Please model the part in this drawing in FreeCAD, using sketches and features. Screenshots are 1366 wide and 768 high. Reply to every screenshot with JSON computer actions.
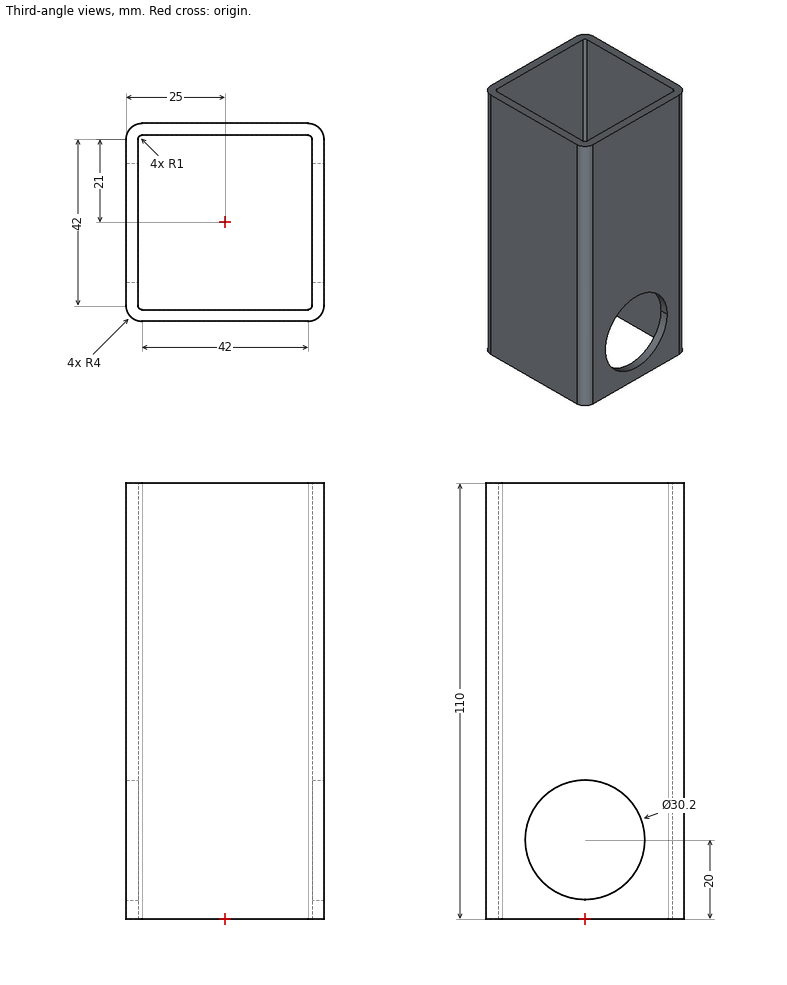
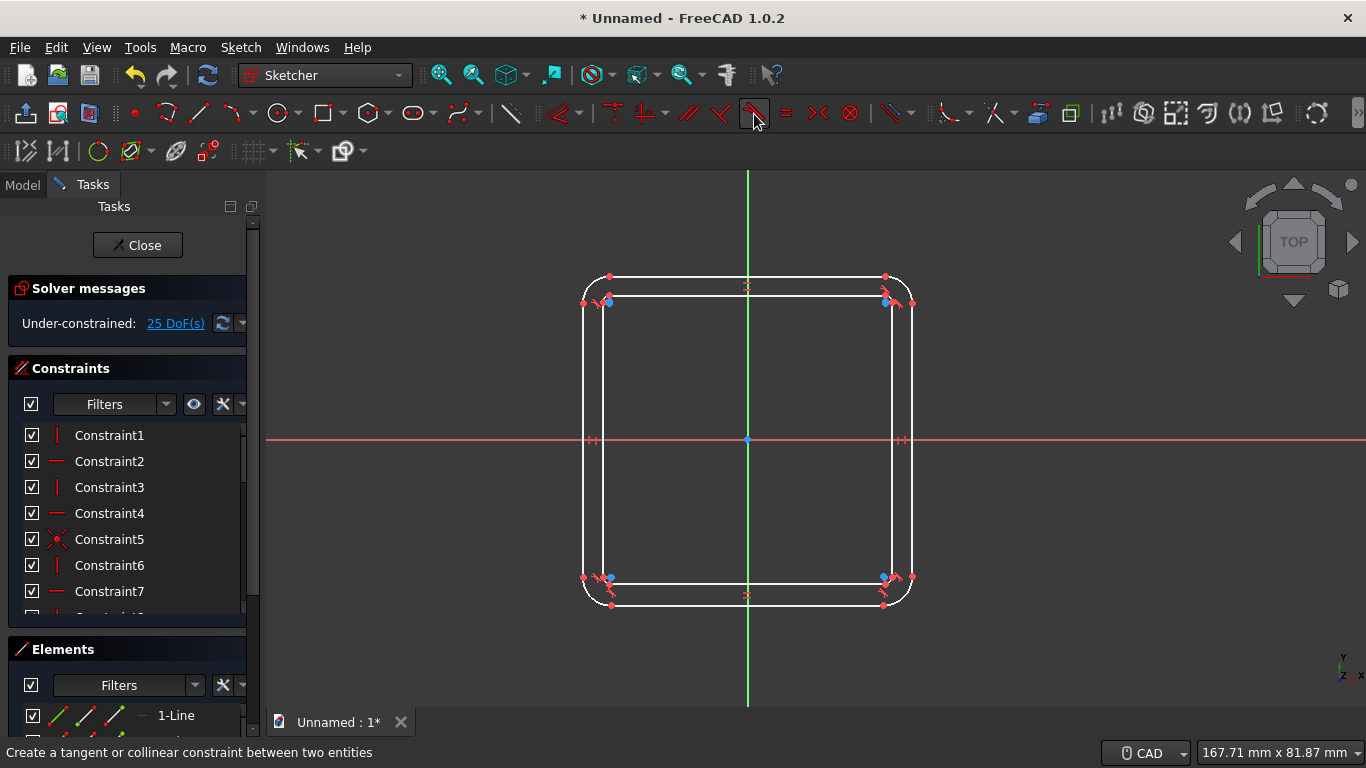
{"action": "left_click", "coordinate": [803, 277]}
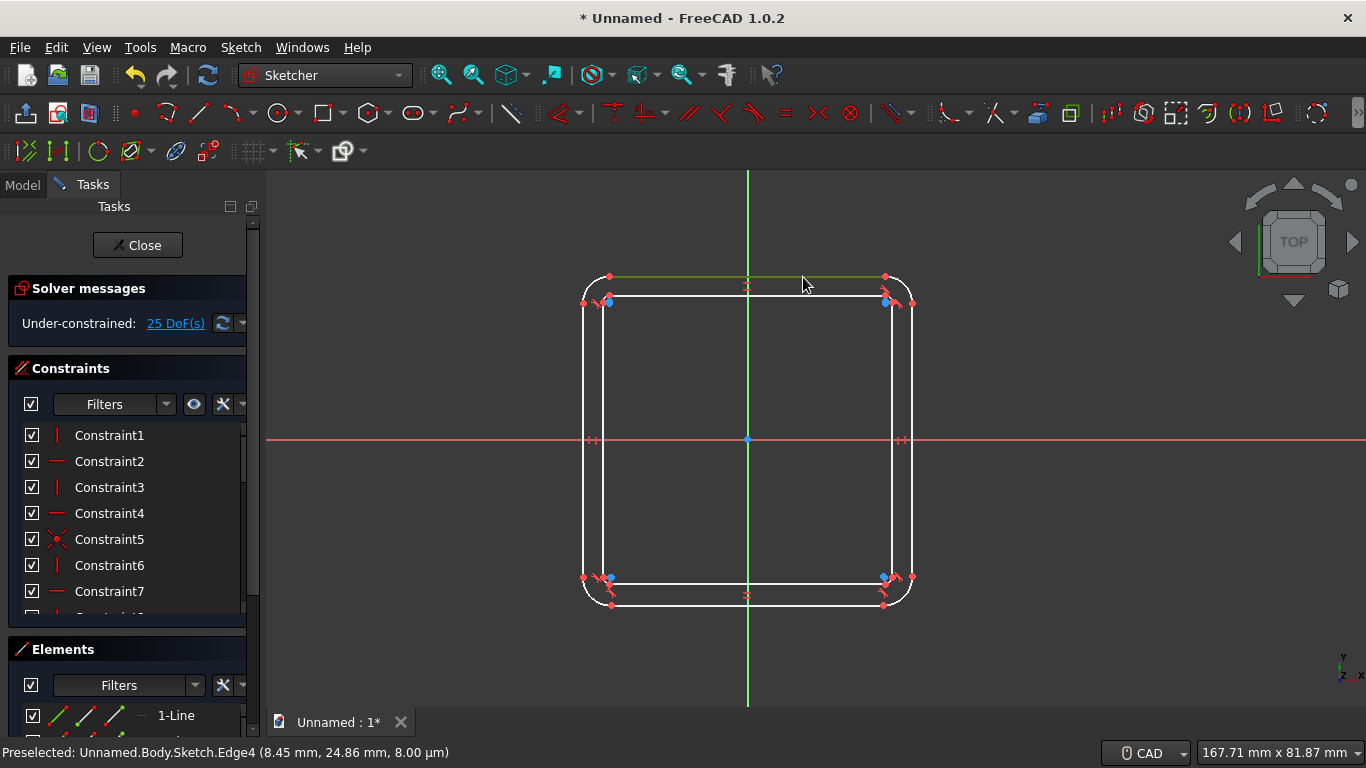
{"action": "left_click", "coordinate": [597, 280]}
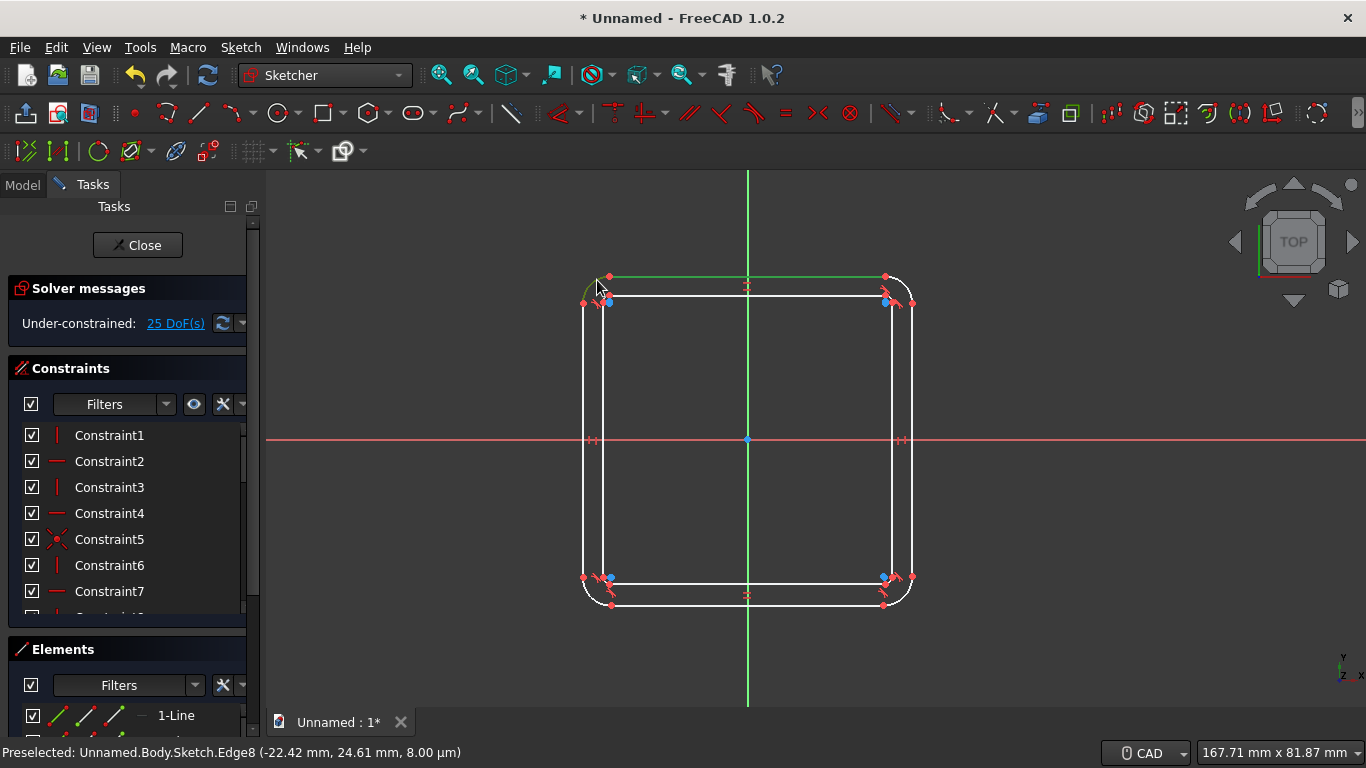
{"action": "left_click", "coordinate": [754, 114]}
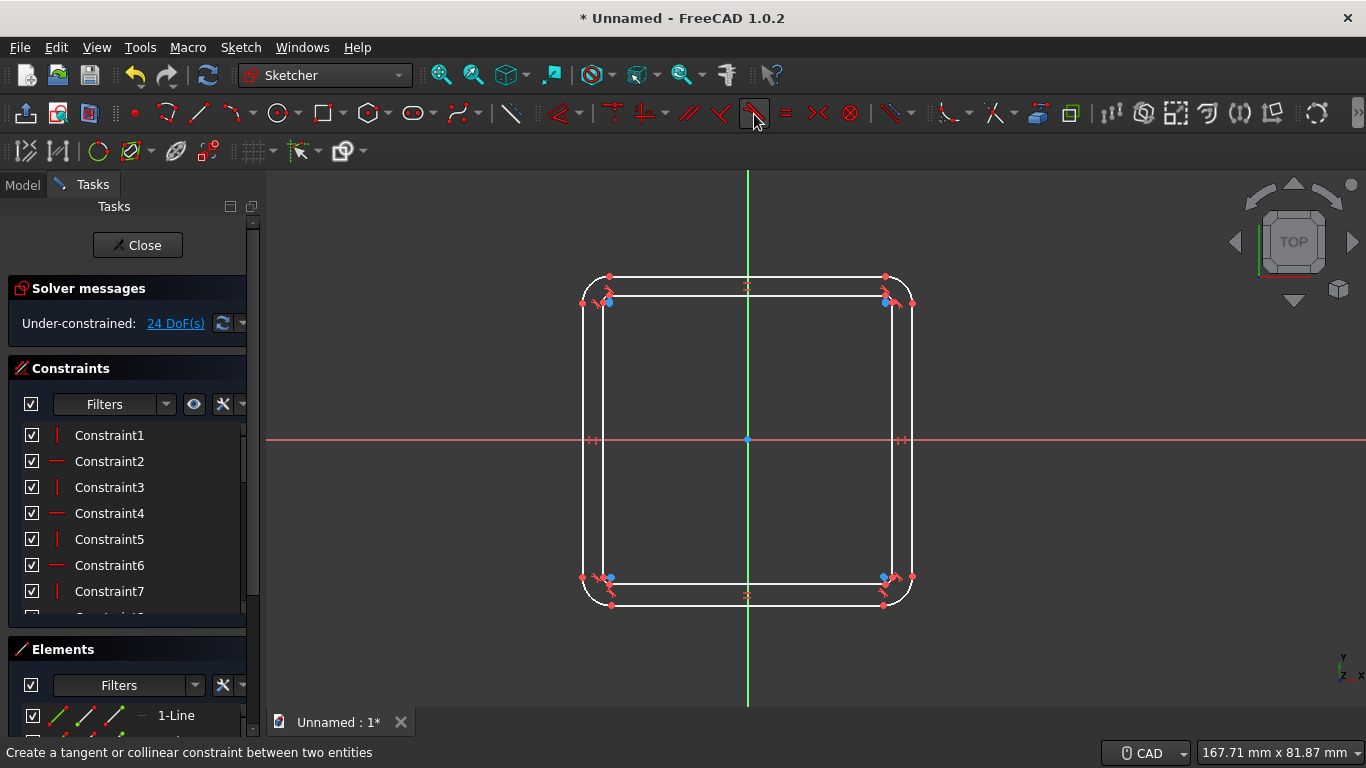
{"action": "left_click", "coordinate": [603, 495]}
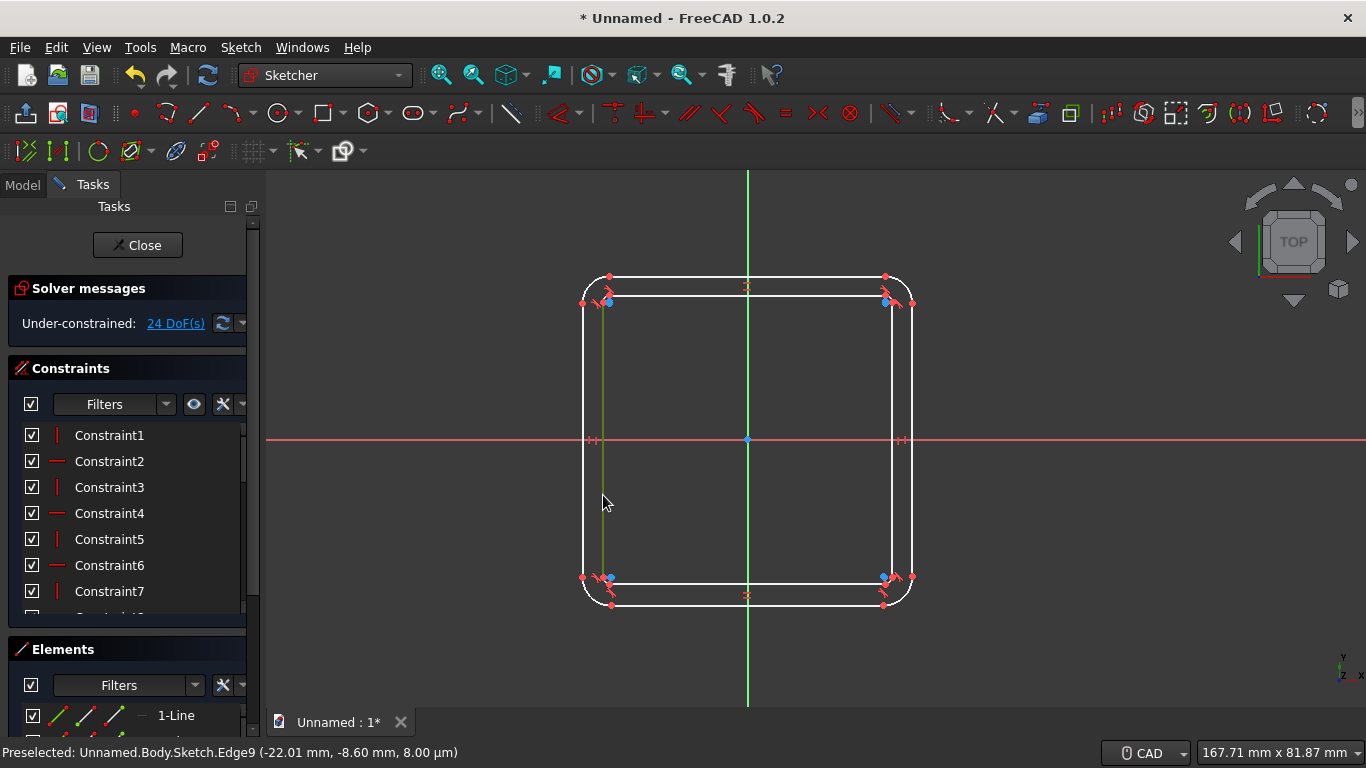
{"action": "scroll", "coordinate": [605, 297], "scroll_direction": "up", "scroll_amount": 5}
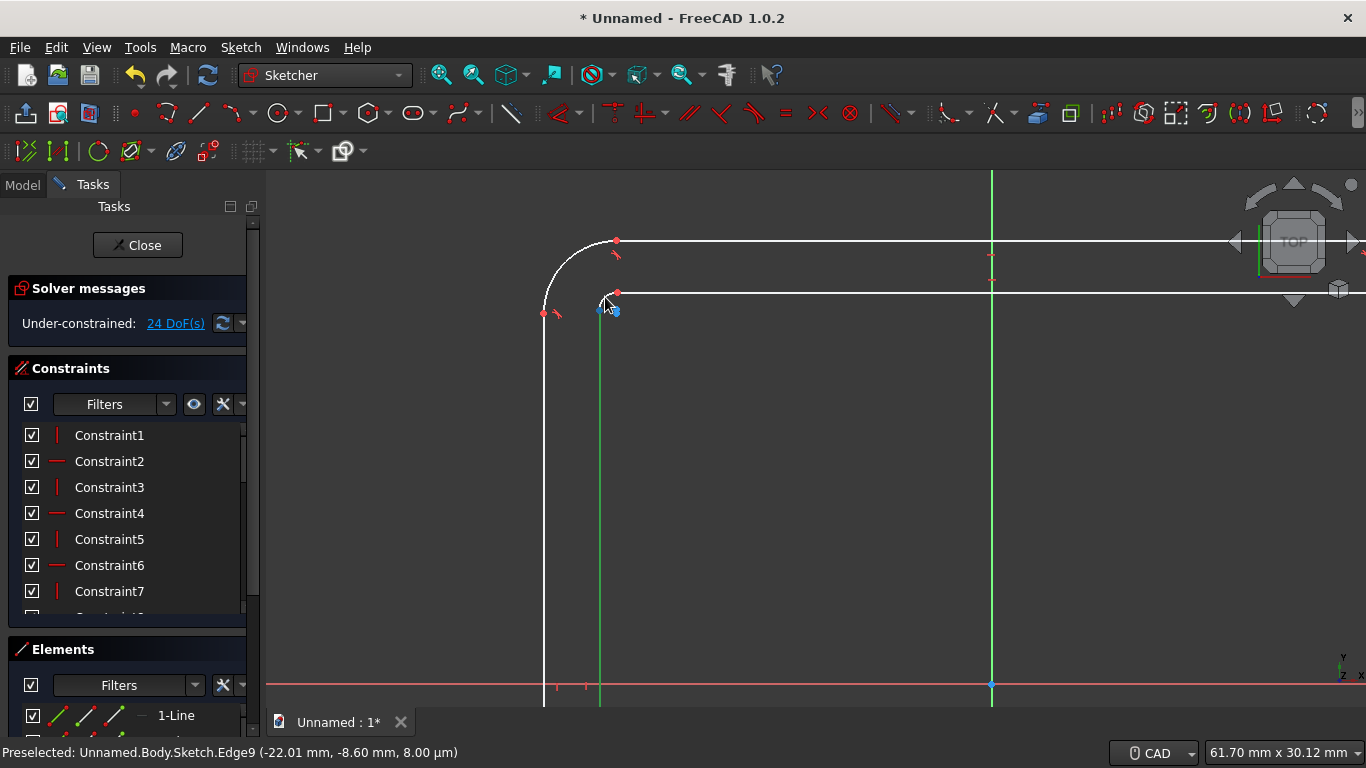
{"action": "left_click", "coordinate": [604, 298]}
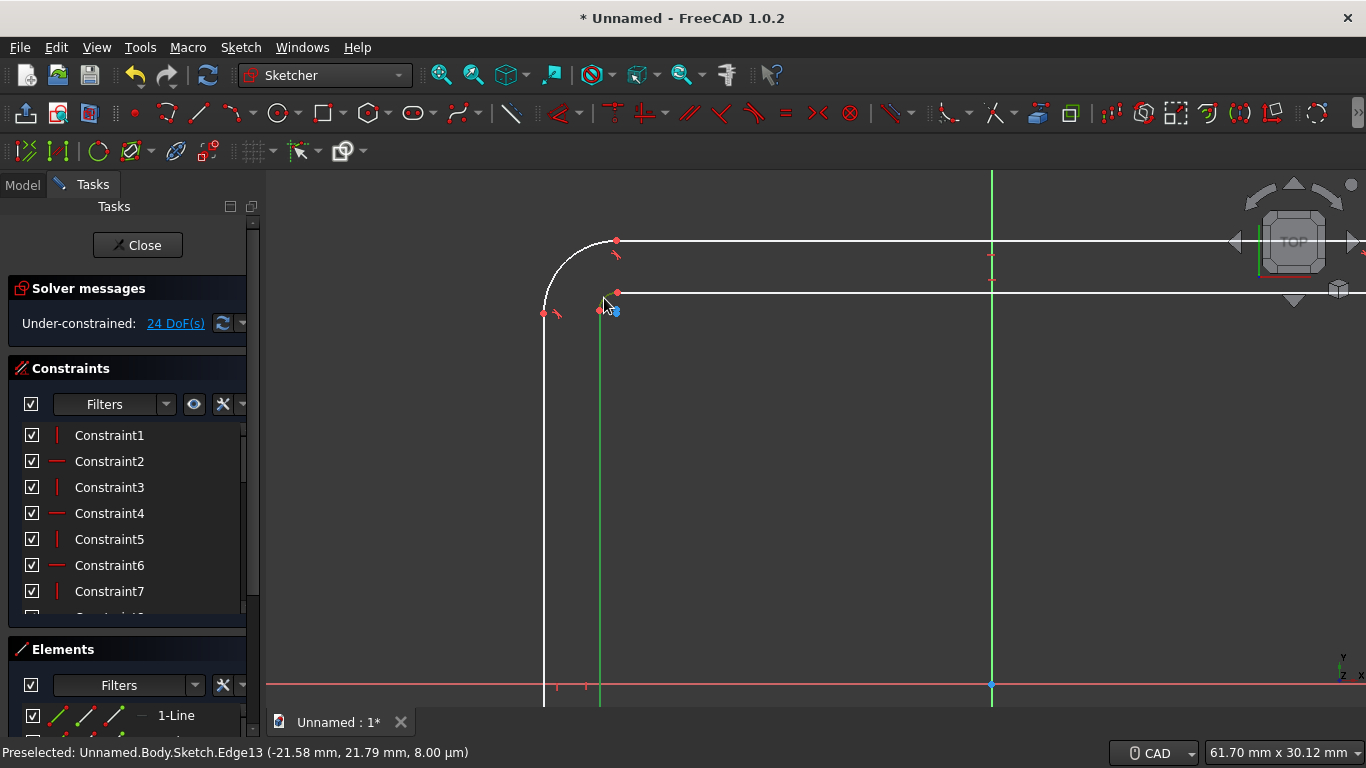
{"action": "left_click", "coordinate": [754, 114]}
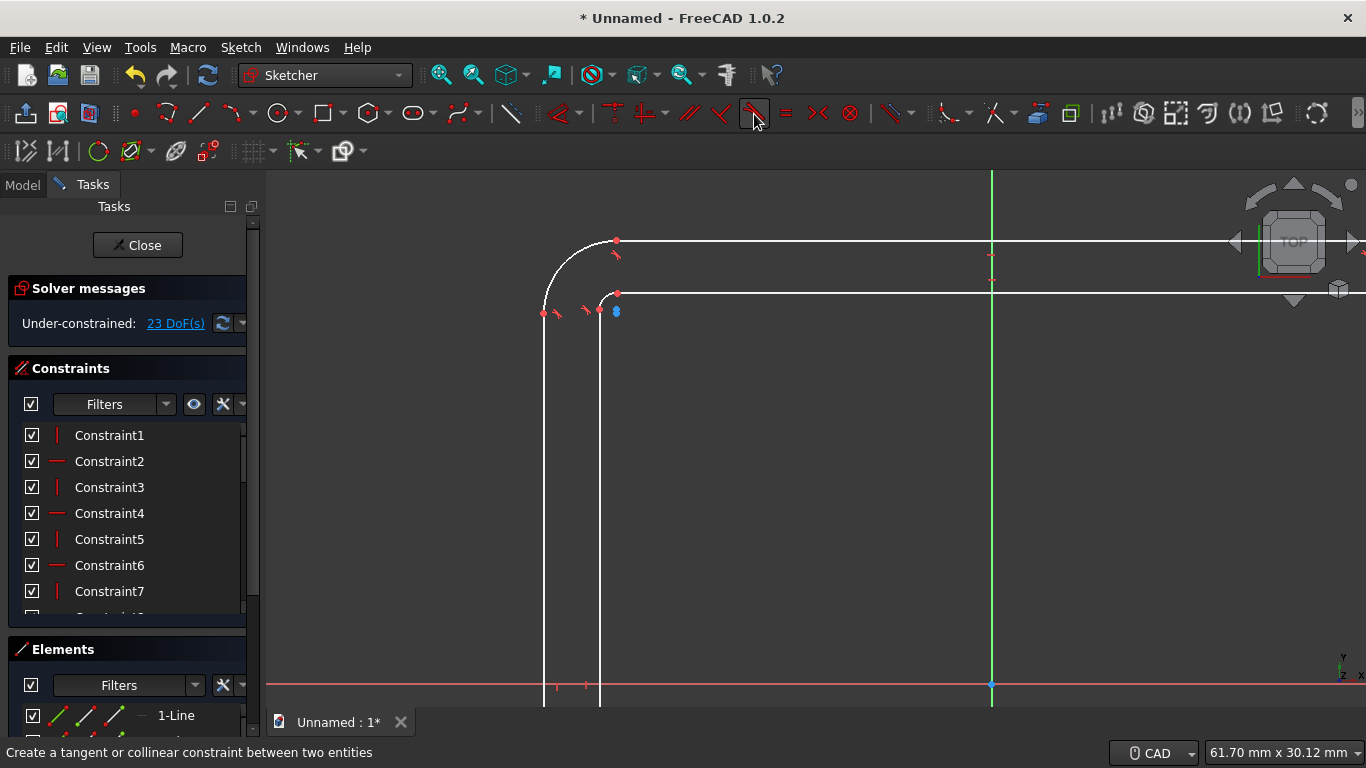
{"action": "left_click", "coordinate": [600, 534]}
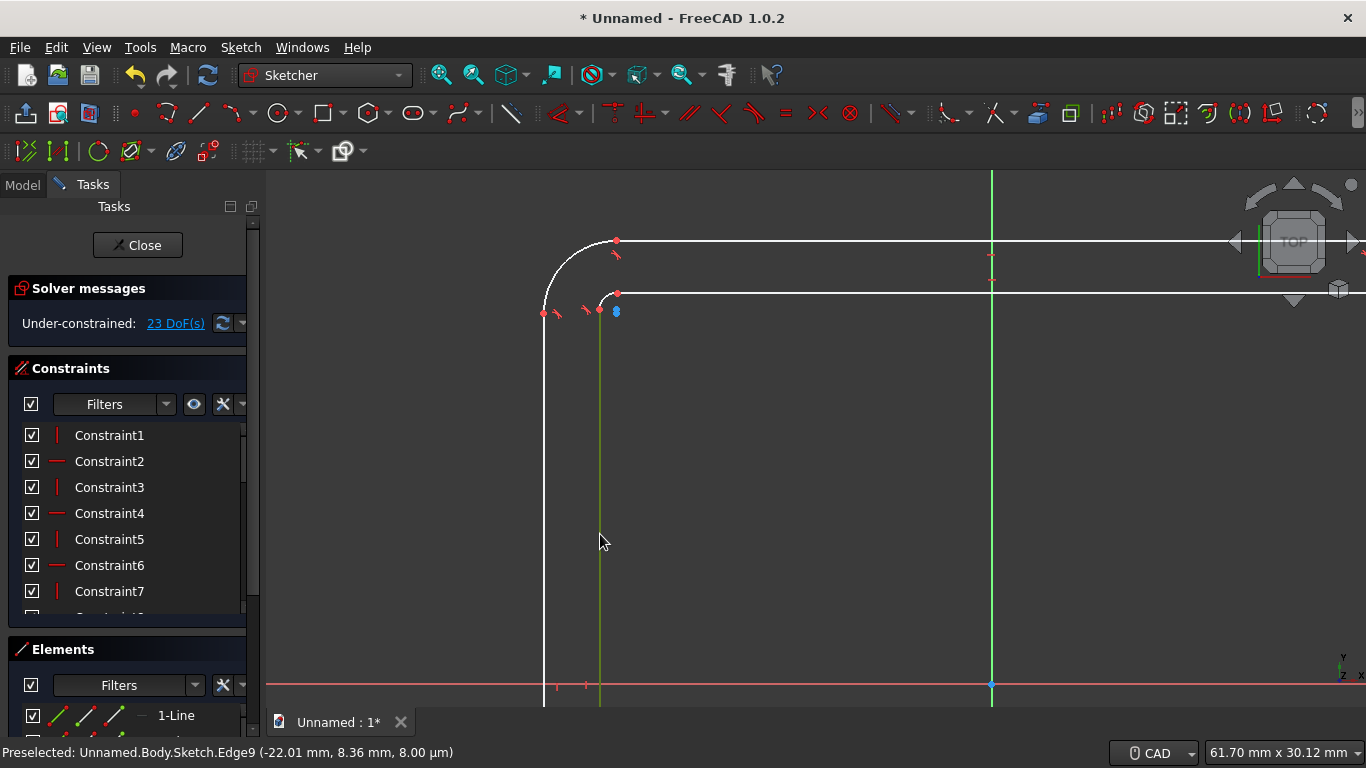
{"action": "scroll", "coordinate": [605, 296], "scroll_direction": "down", "scroll_amount": 5}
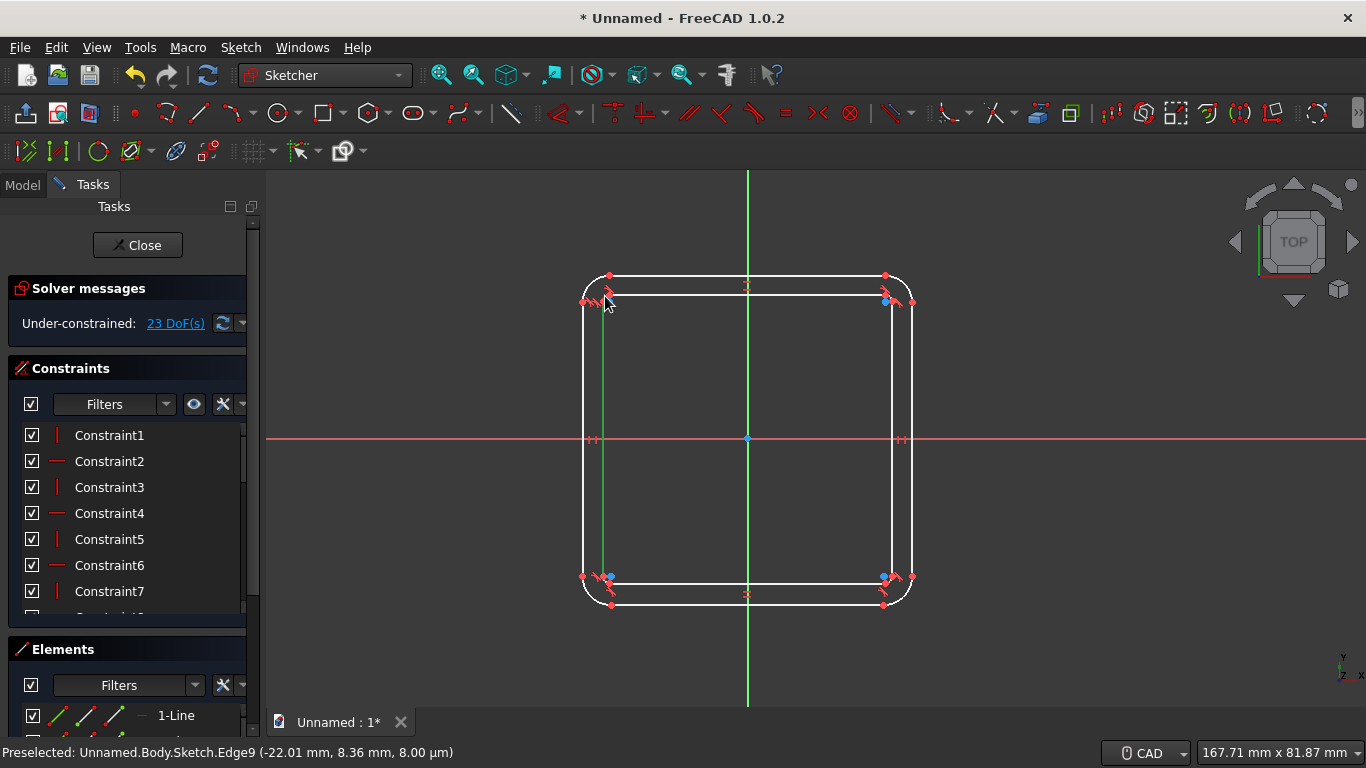
{"action": "scroll", "coordinate": [605, 582], "scroll_direction": "up", "scroll_amount": 6}